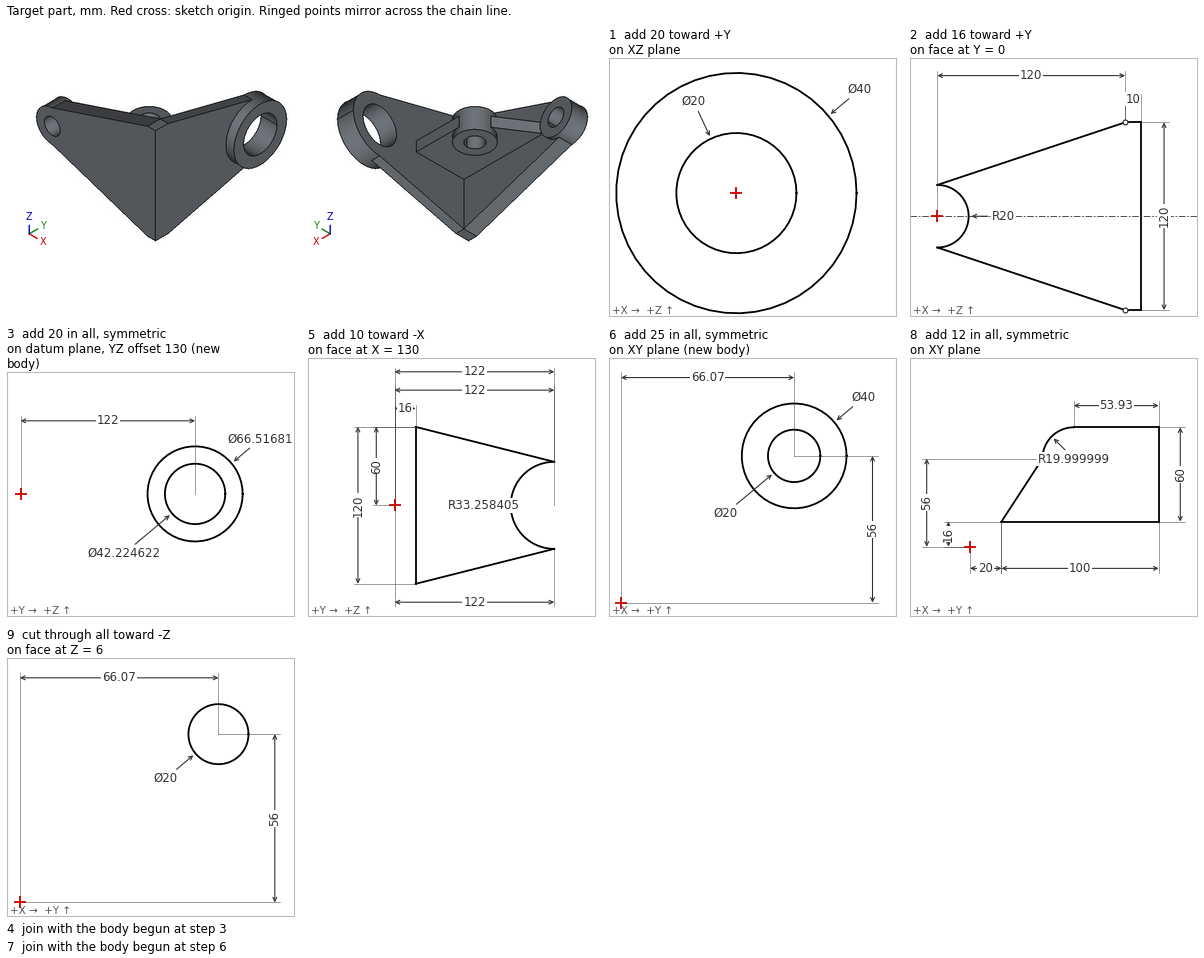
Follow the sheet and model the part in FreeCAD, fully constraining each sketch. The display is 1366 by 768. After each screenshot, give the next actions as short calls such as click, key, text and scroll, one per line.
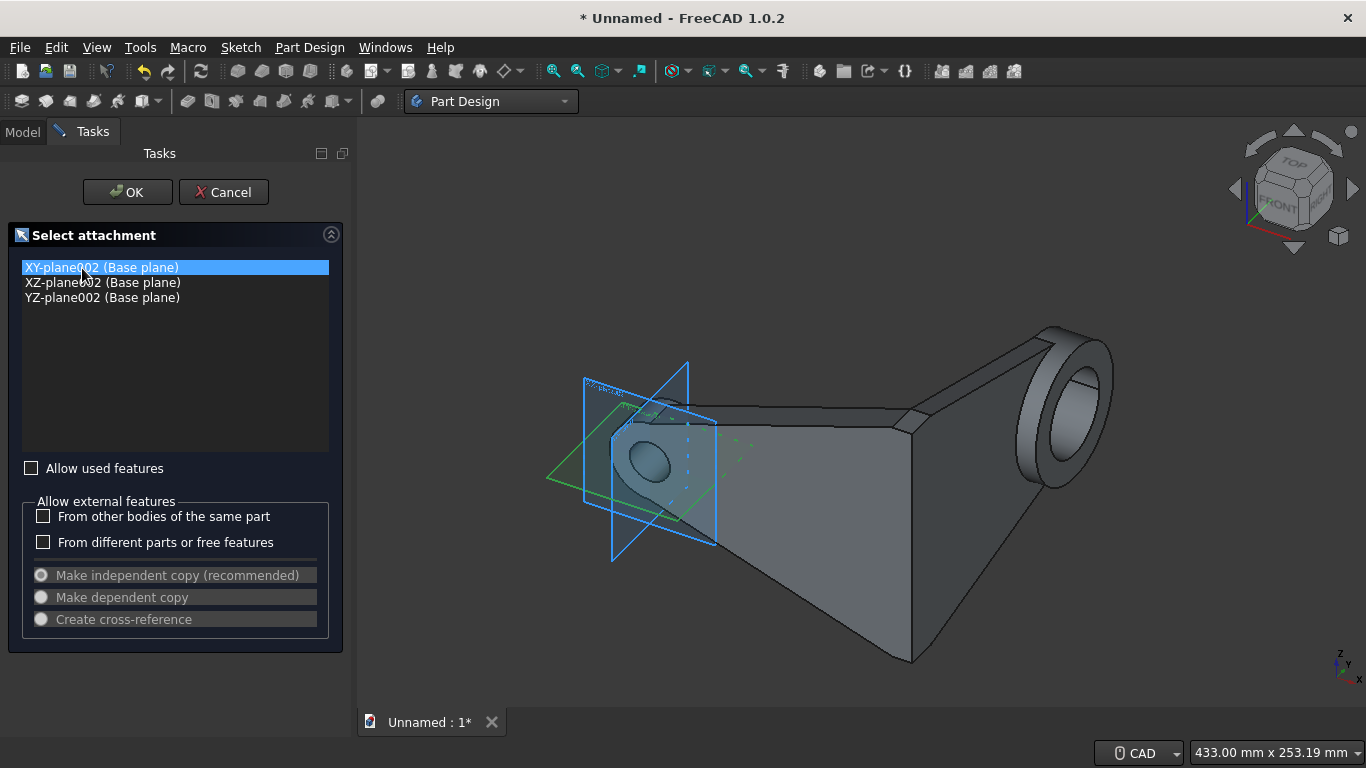
click(128, 192)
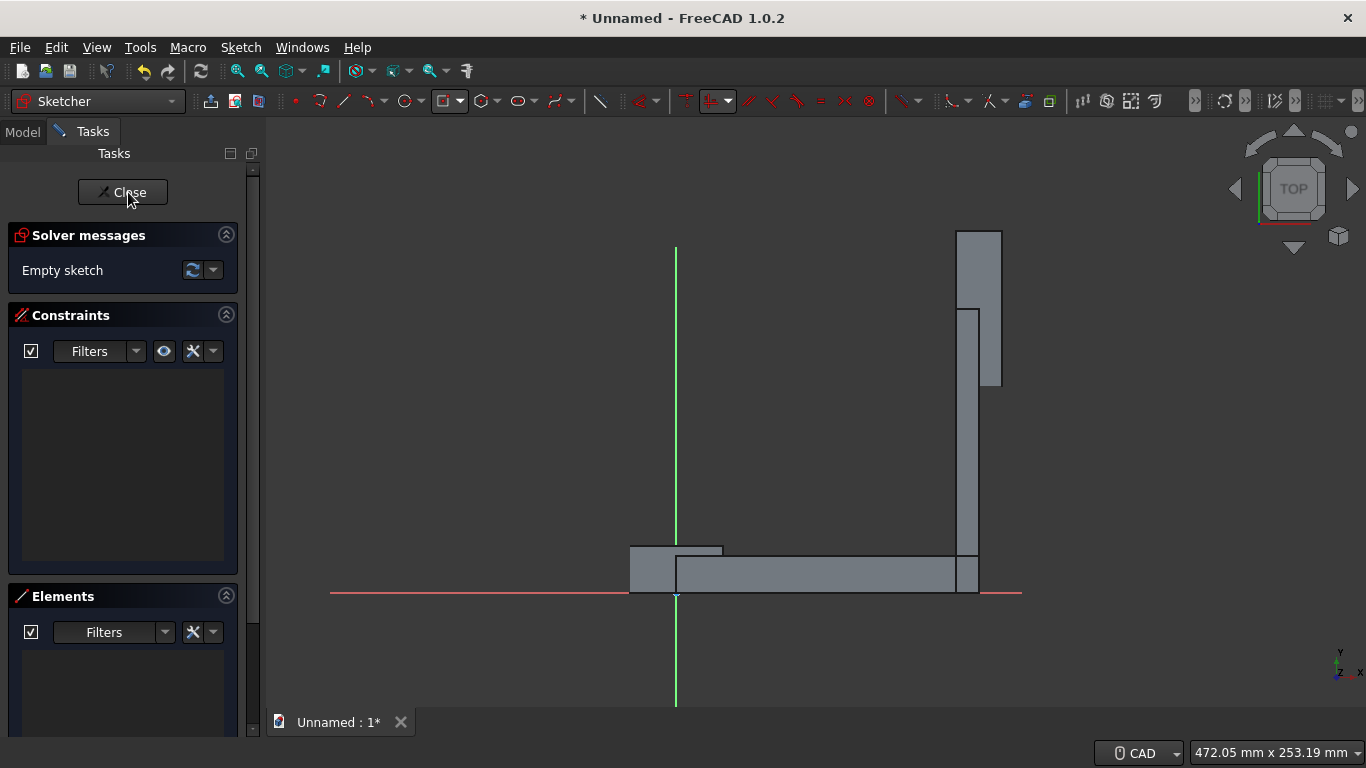
scroll(800, 580, up, 4)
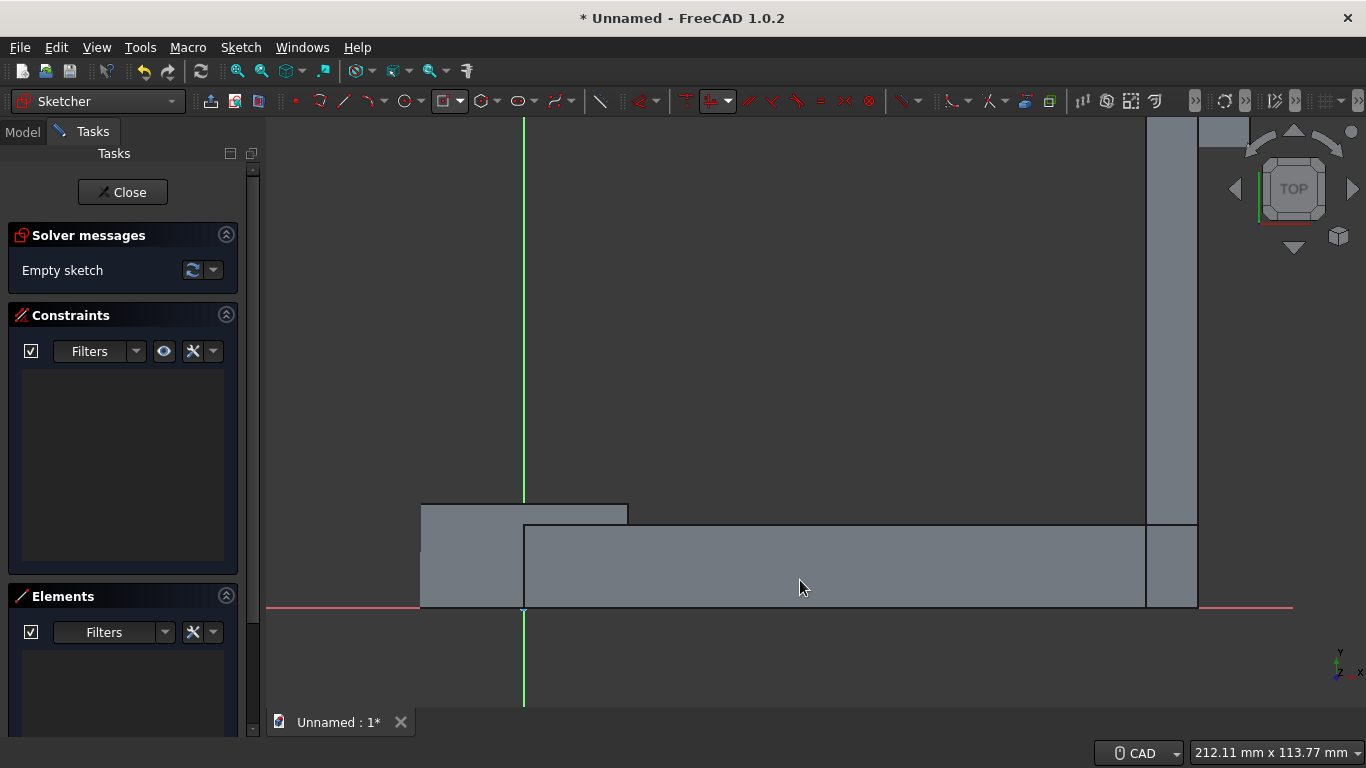
click(406, 102)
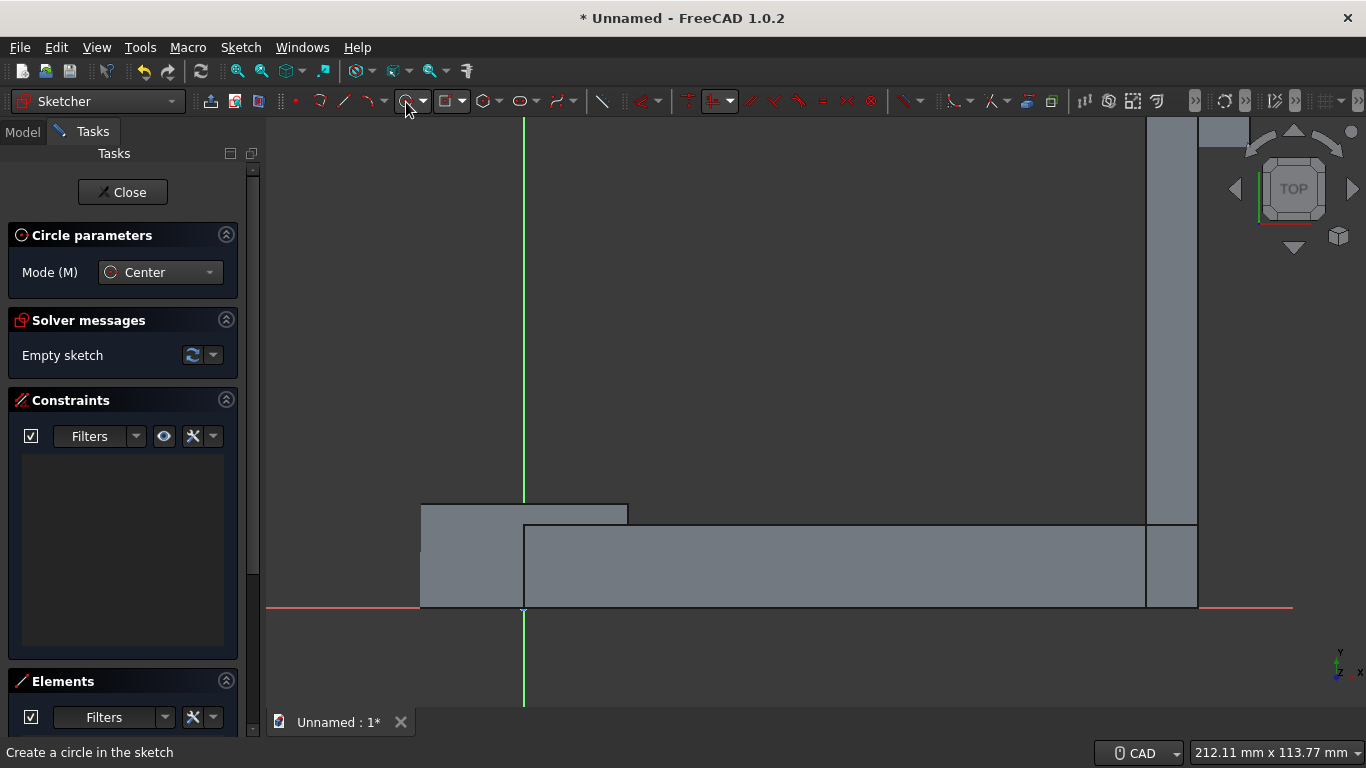
click(866, 317)
click(940, 244)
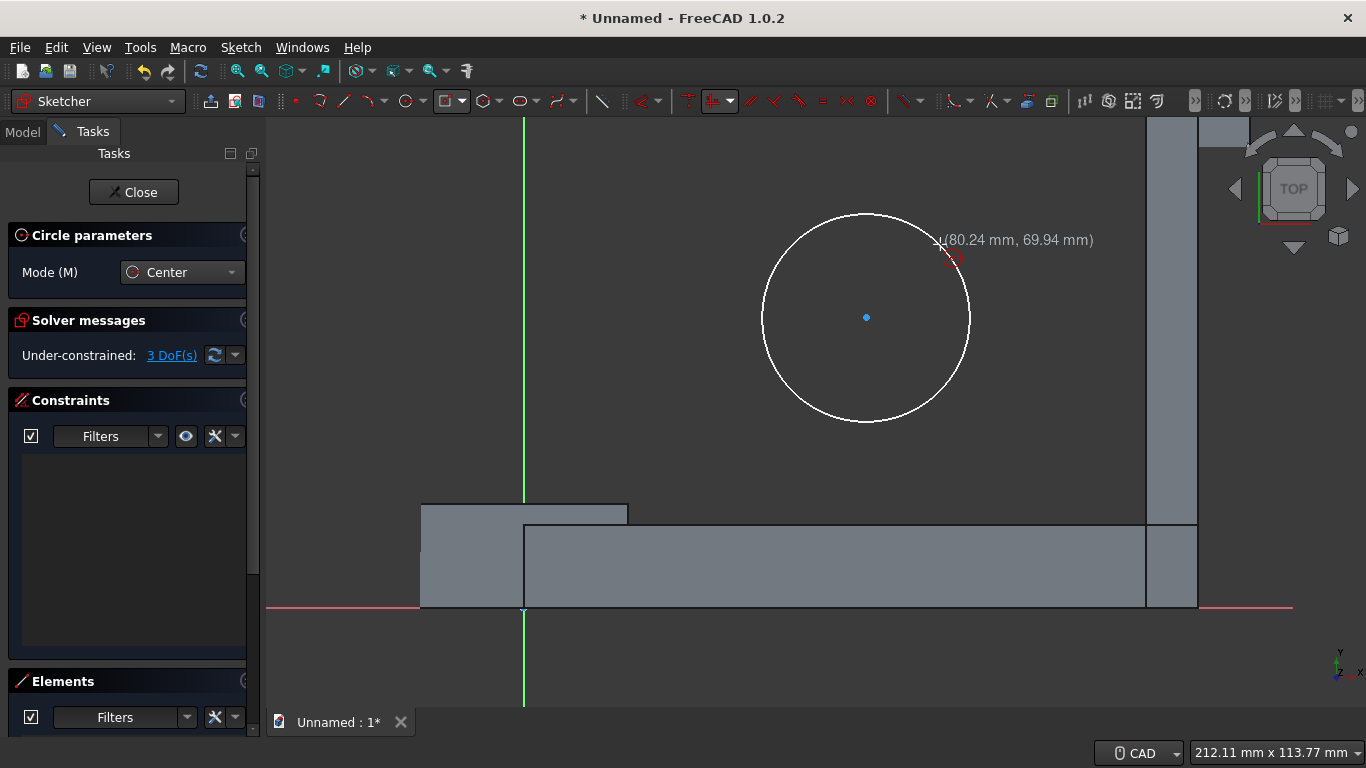
click(866, 318)
click(903, 281)
key(Escape)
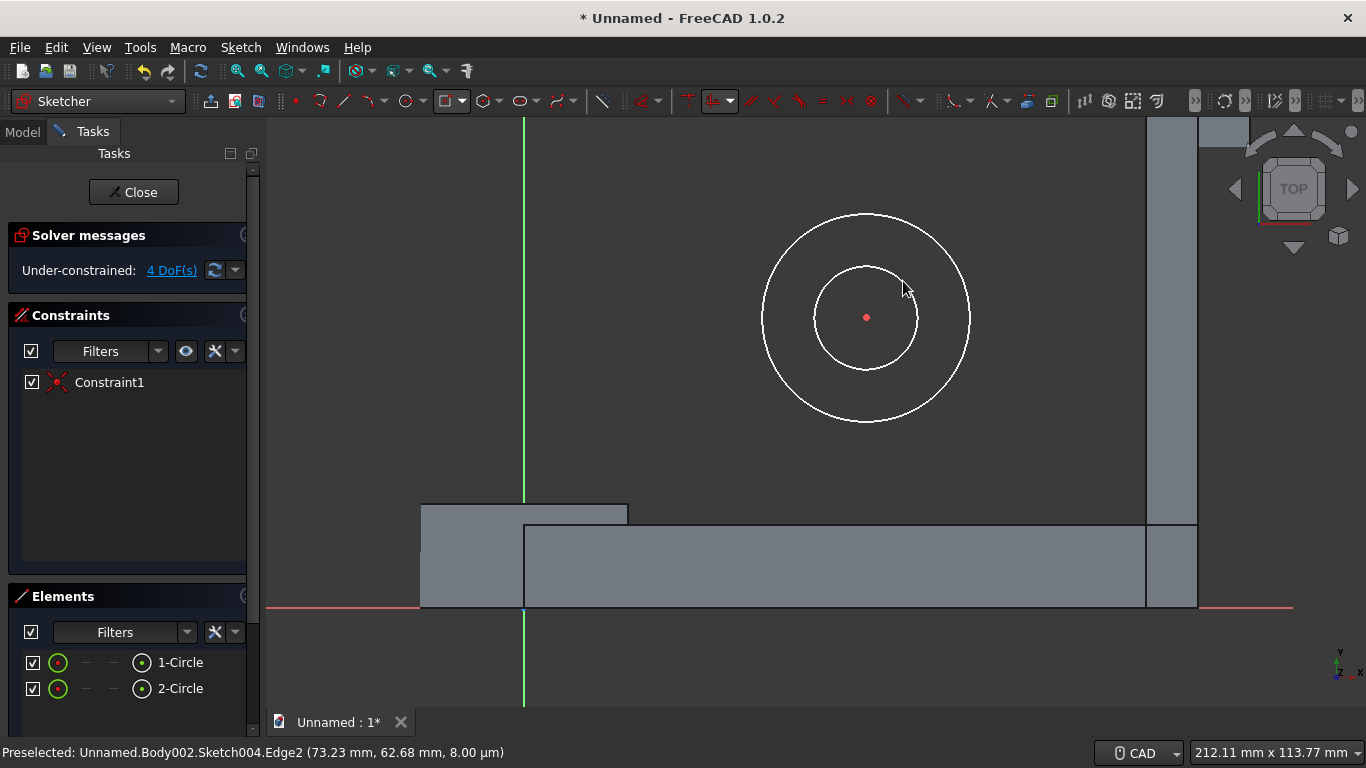
click(642, 102)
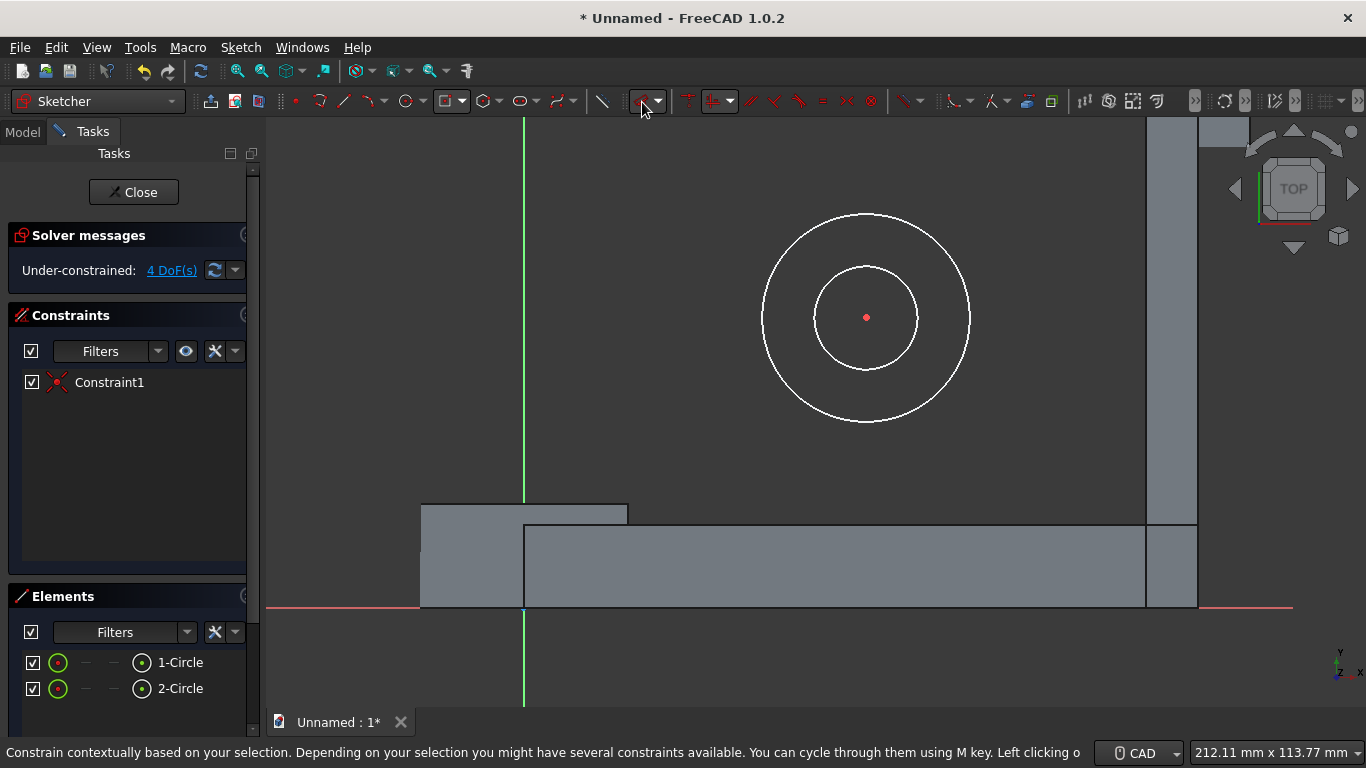
click(939, 244)
click(961, 221)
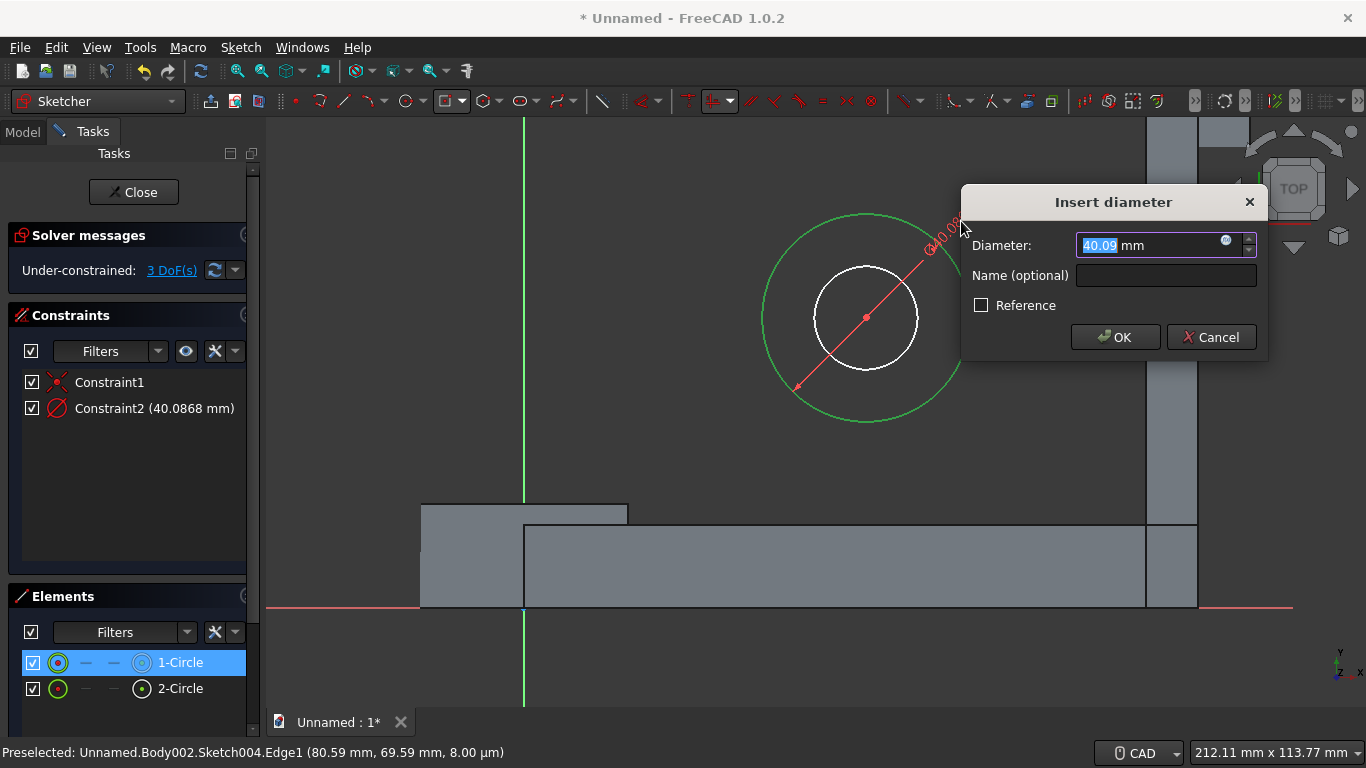
text(40)
key(Return)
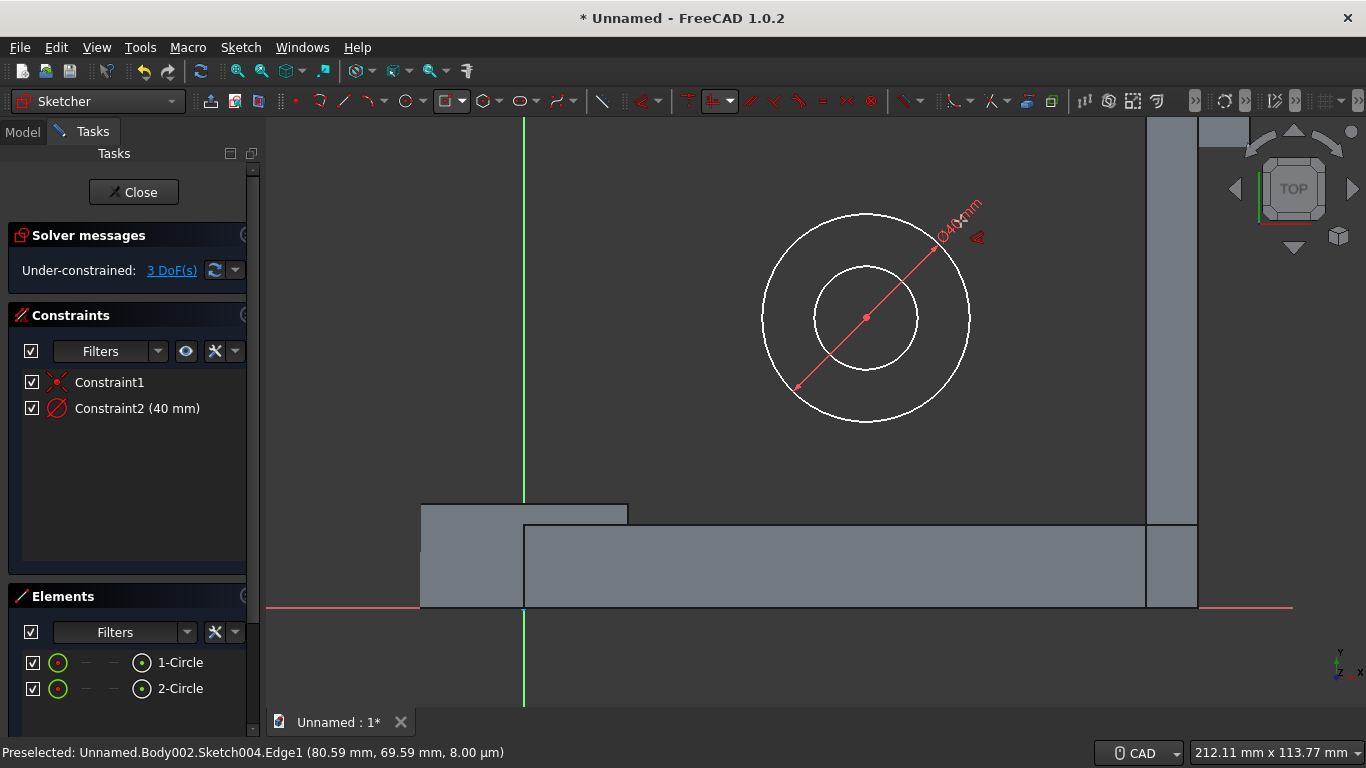
click(902, 281)
click(924, 258)